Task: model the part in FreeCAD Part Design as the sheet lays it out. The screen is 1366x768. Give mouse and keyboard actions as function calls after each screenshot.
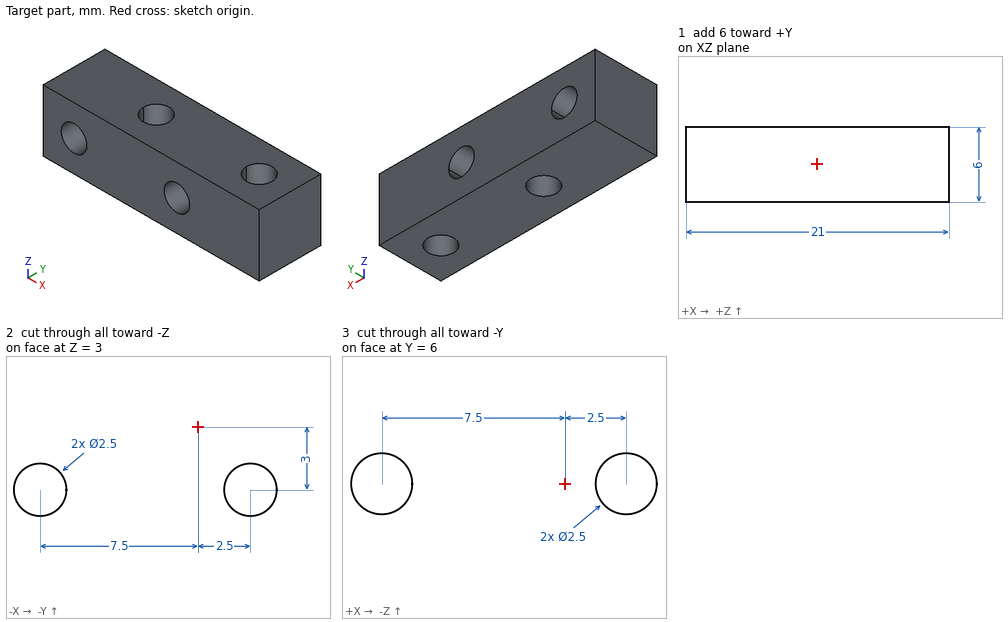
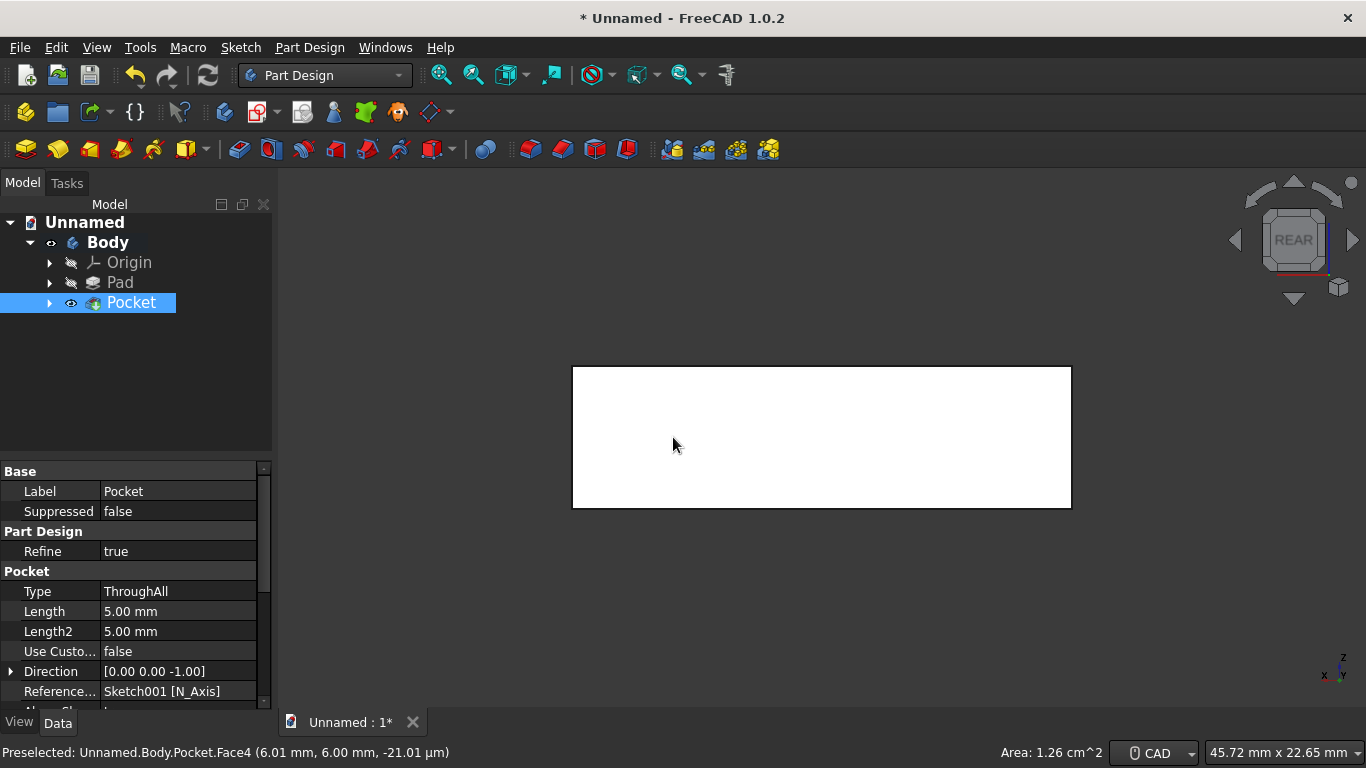
click(258, 112)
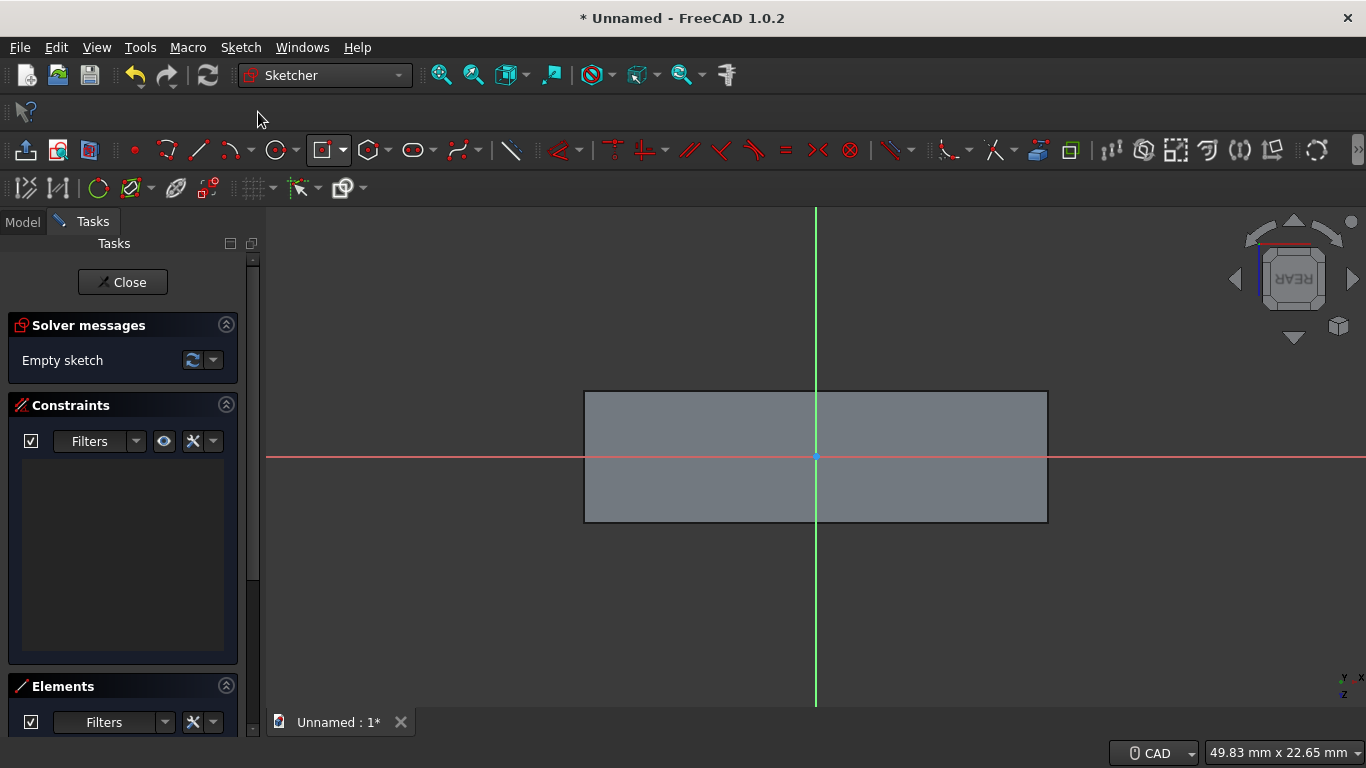
scroll(772, 457, up, 4)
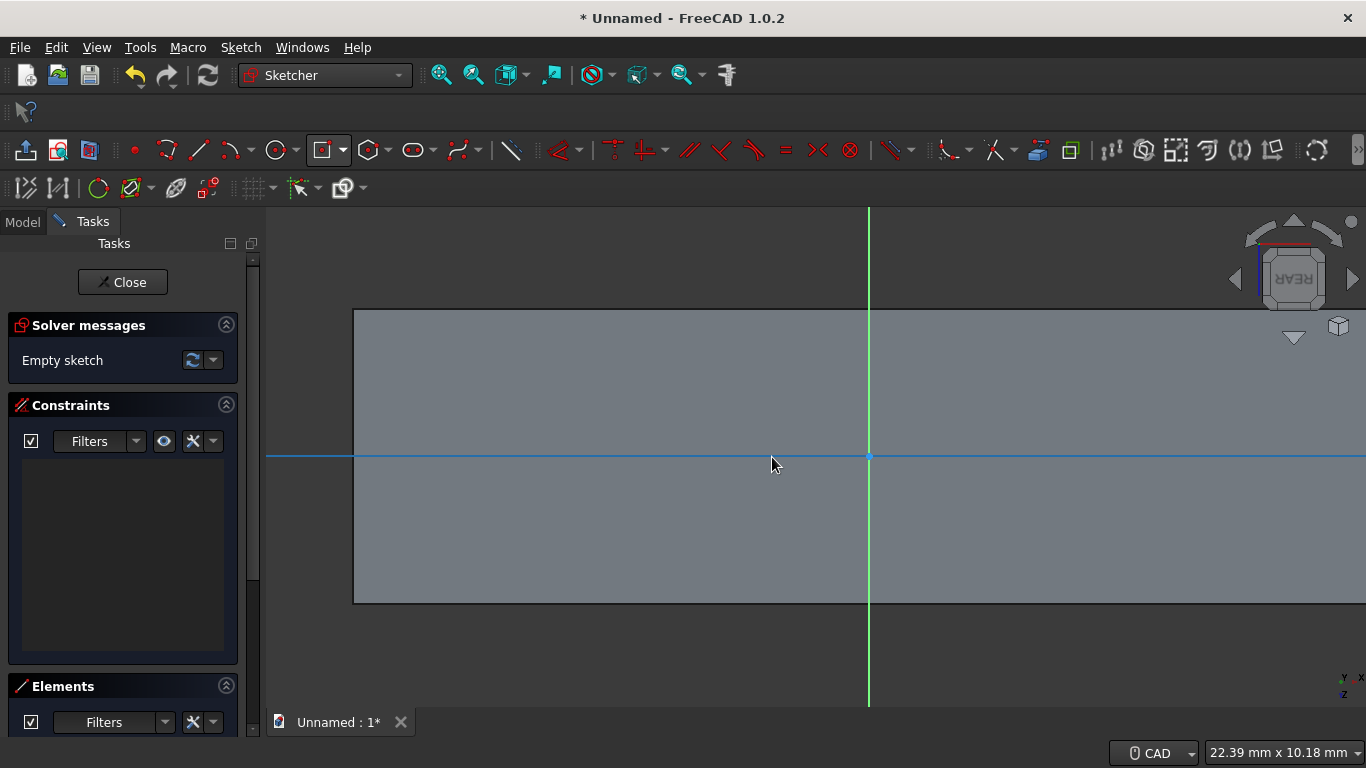
click(276, 150)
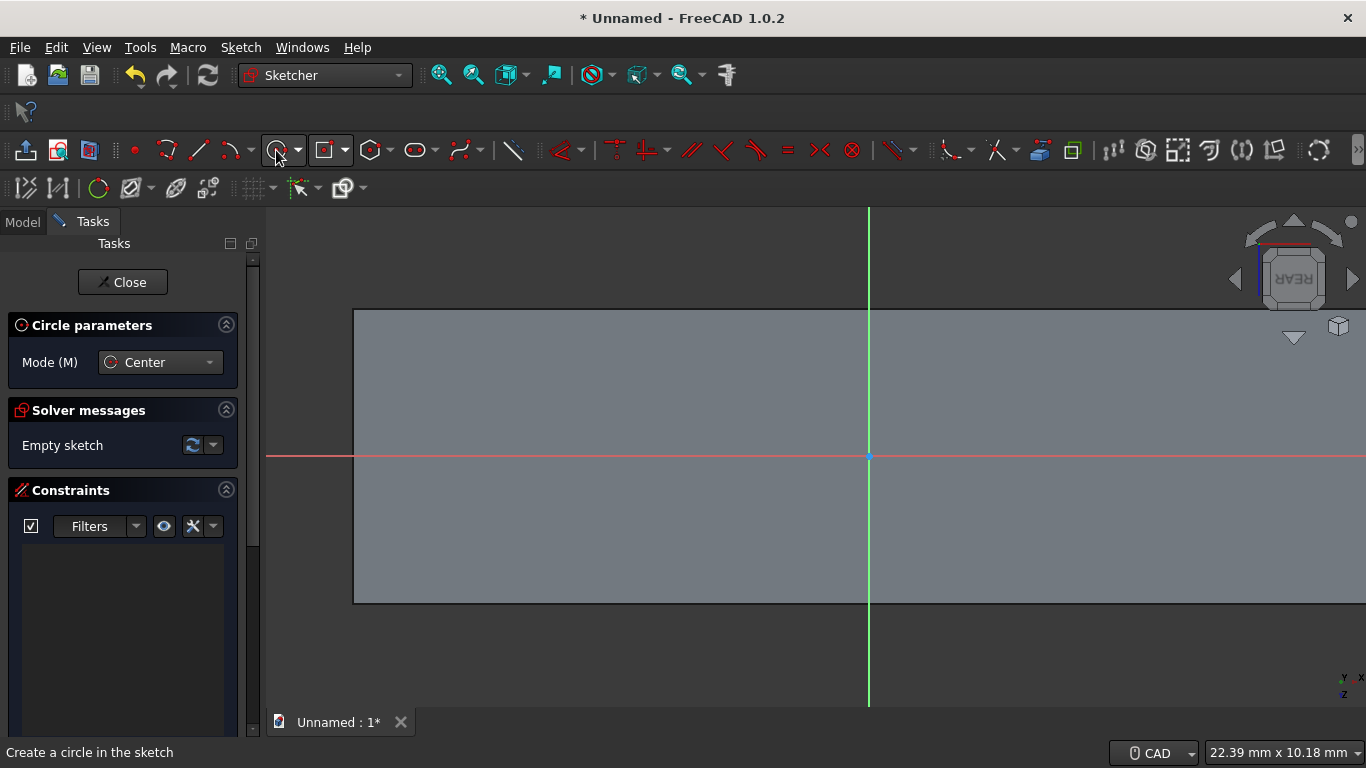
click(992, 456)
move(1036, 413)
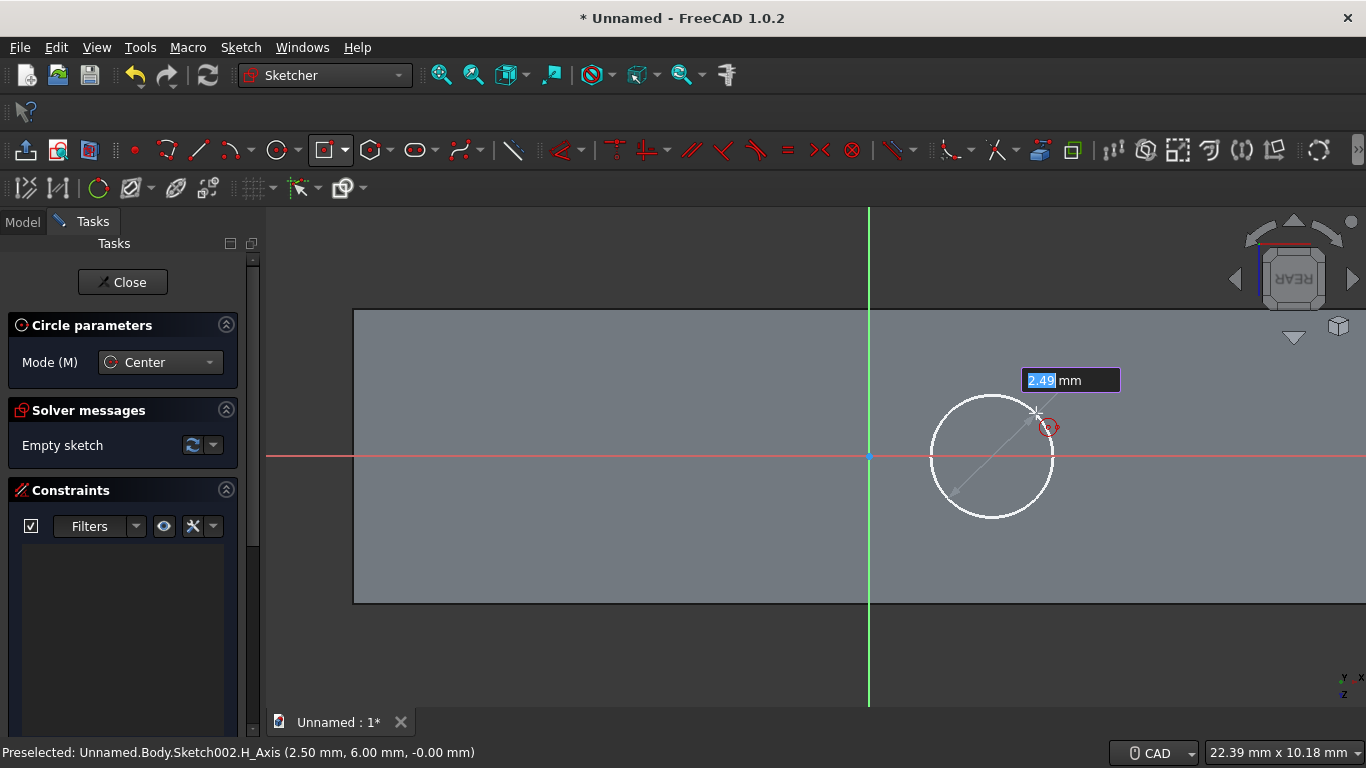
text(2.5)
key(Return)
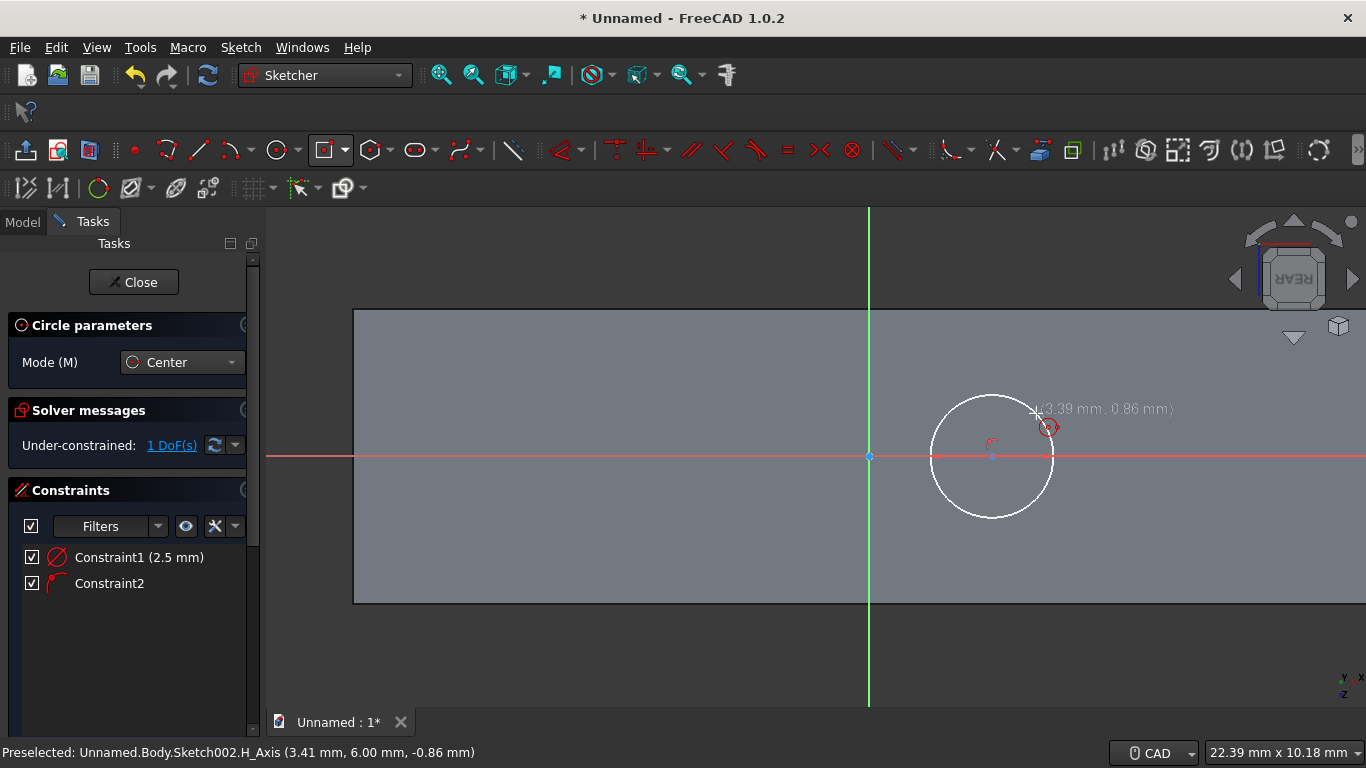
click(501, 456)
move(544, 413)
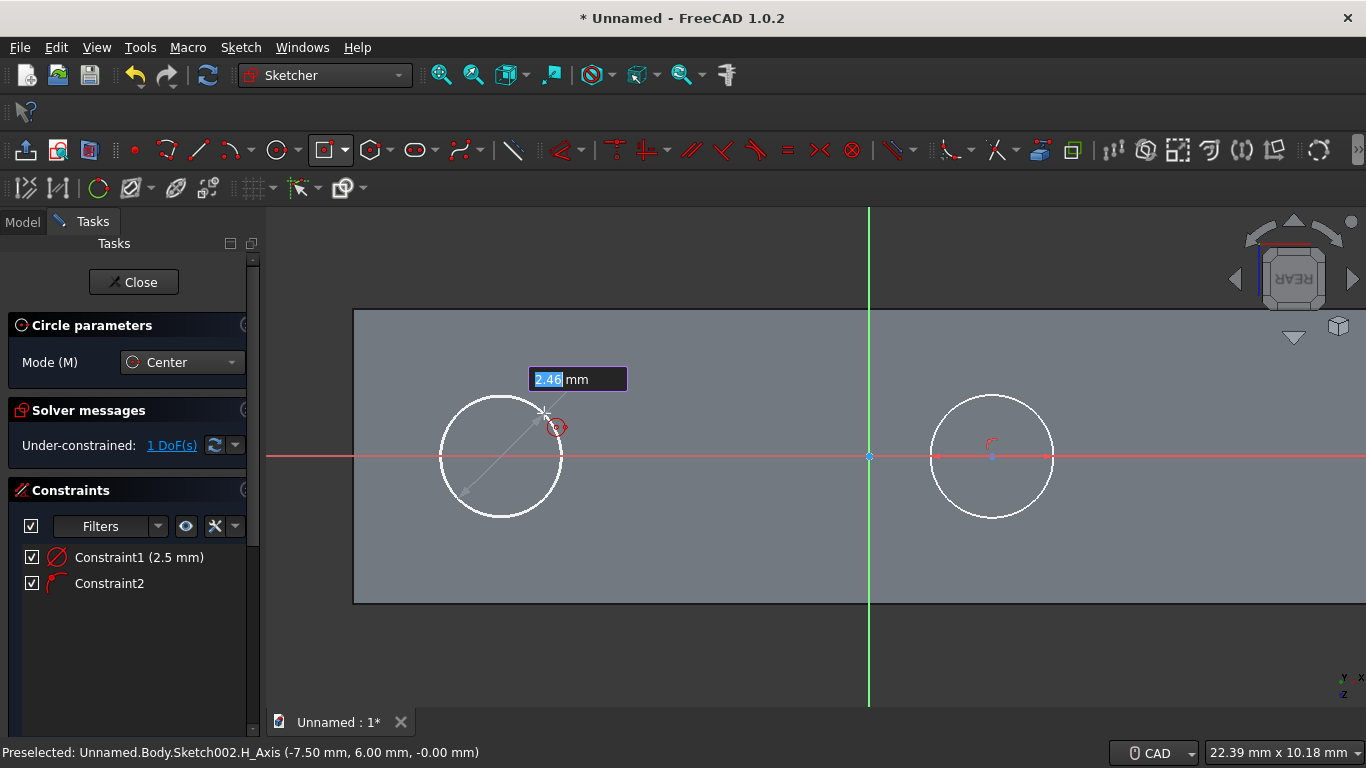
text(2.5)
key(Return)
key(Escape)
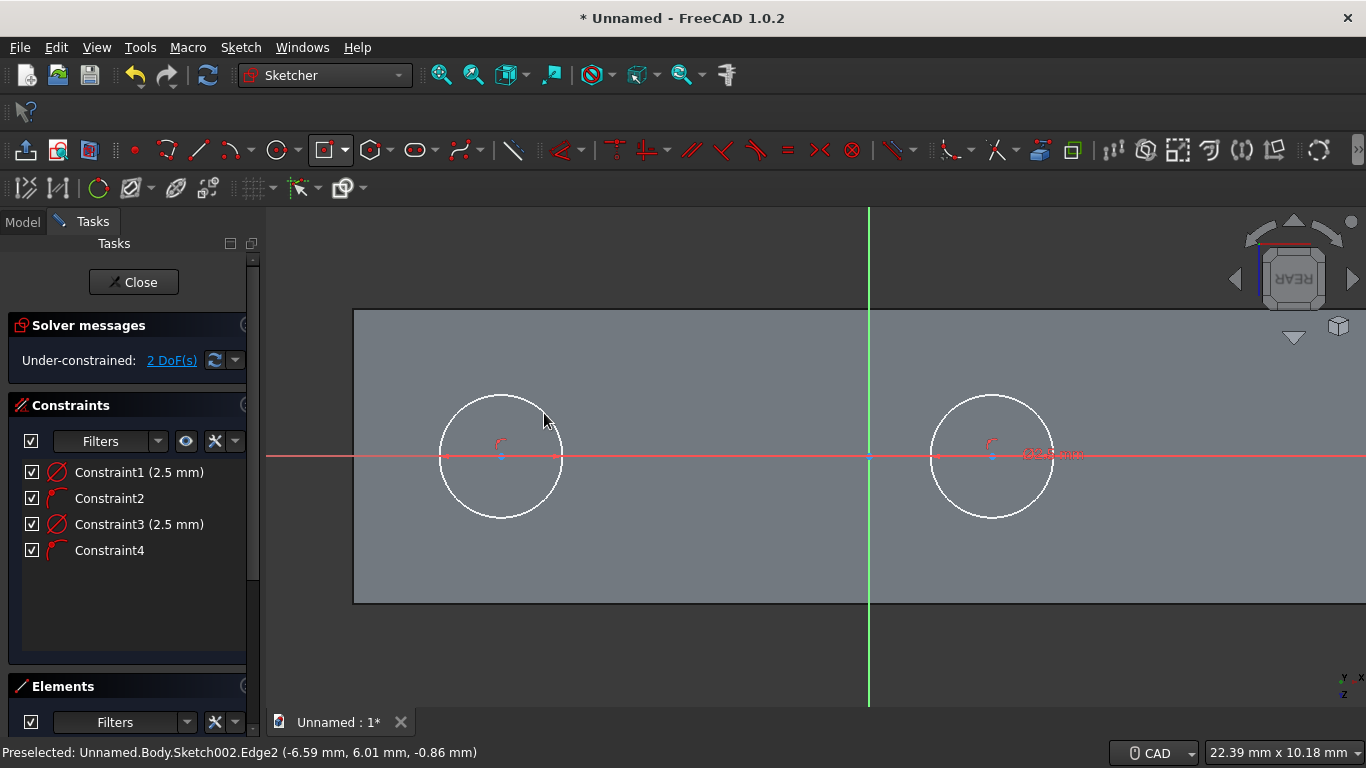
click(560, 150)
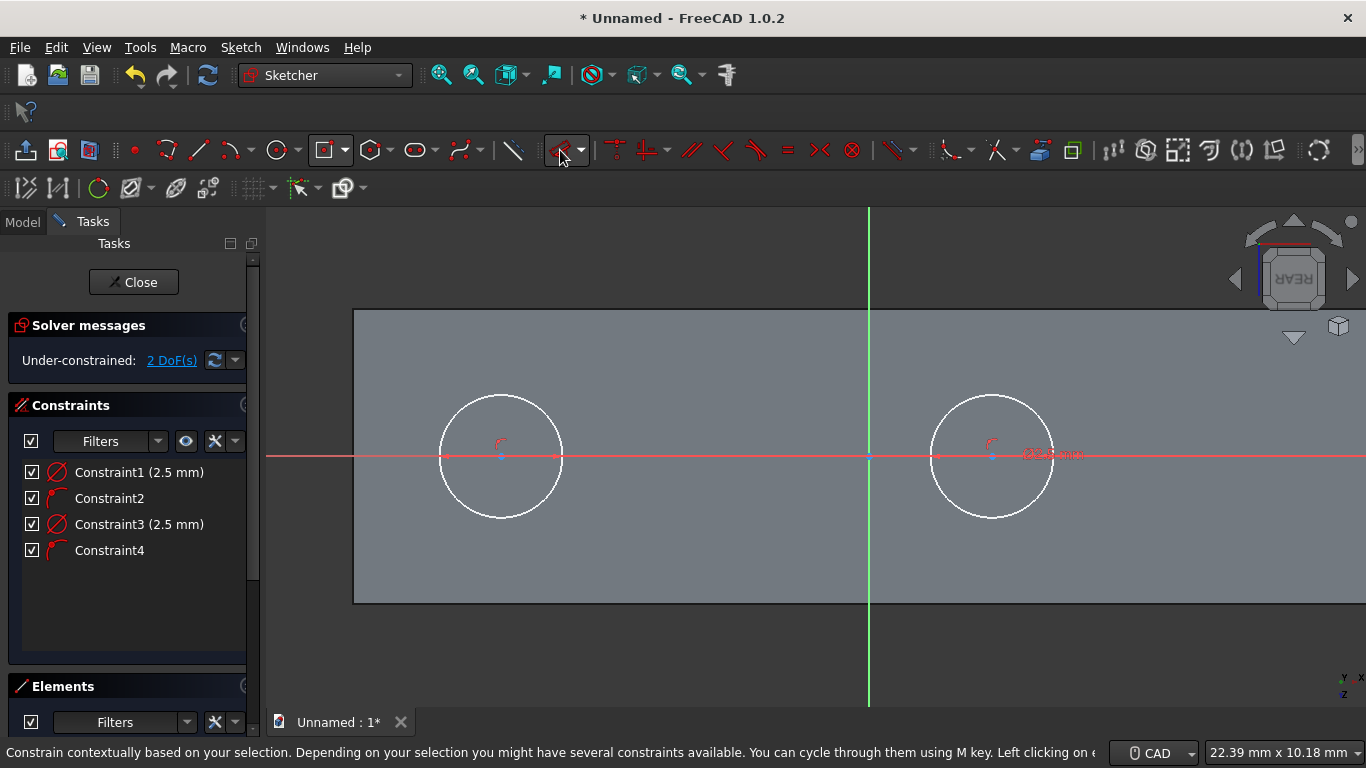
click(992, 456)
click(902, 490)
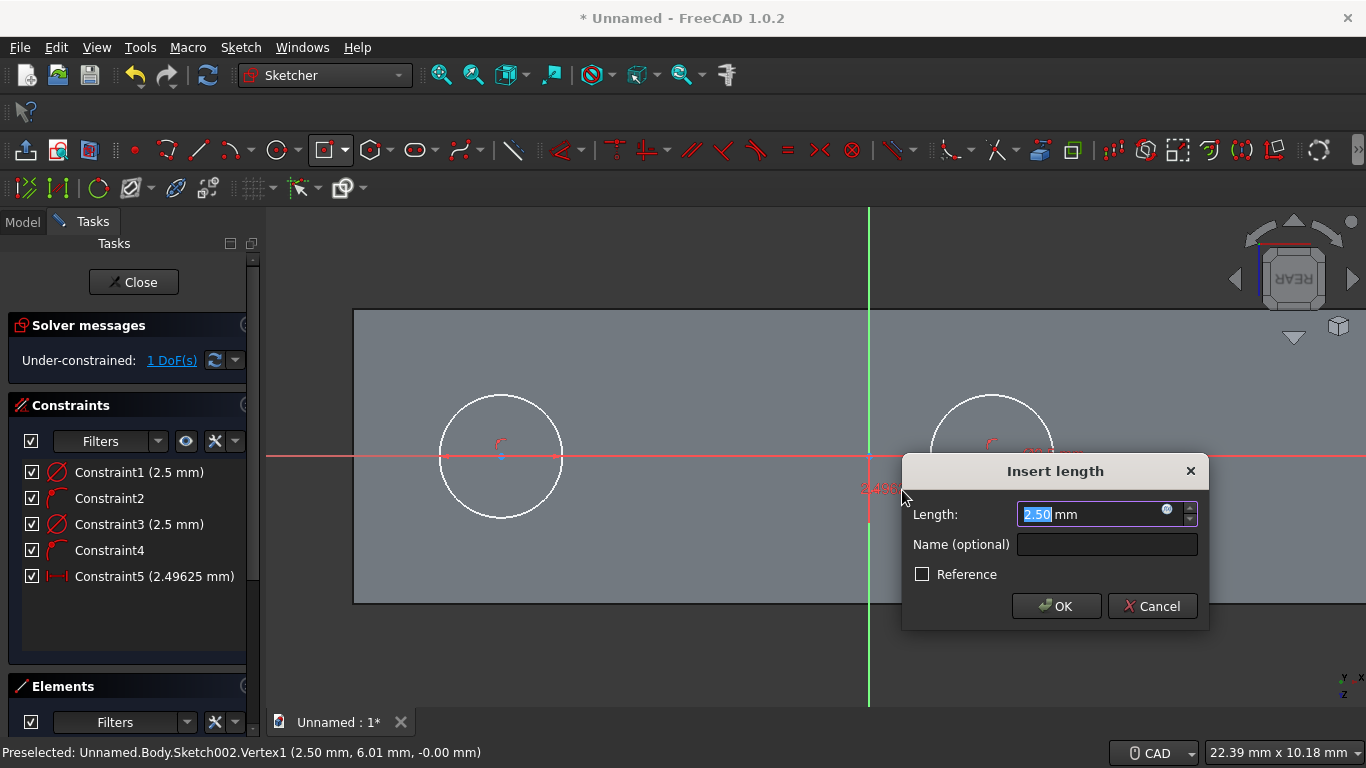
text(2.5)
key(Return)